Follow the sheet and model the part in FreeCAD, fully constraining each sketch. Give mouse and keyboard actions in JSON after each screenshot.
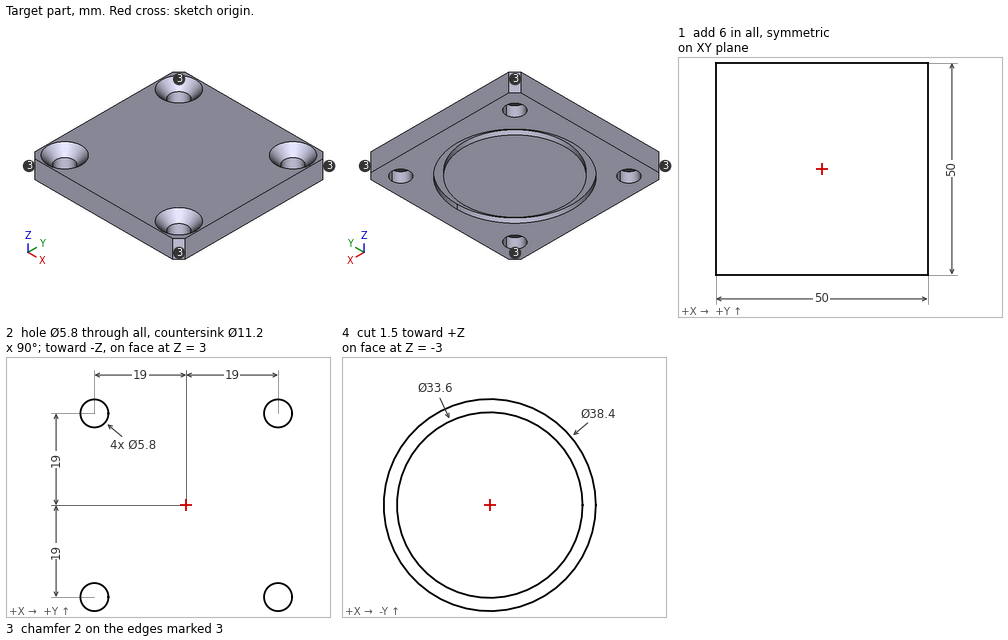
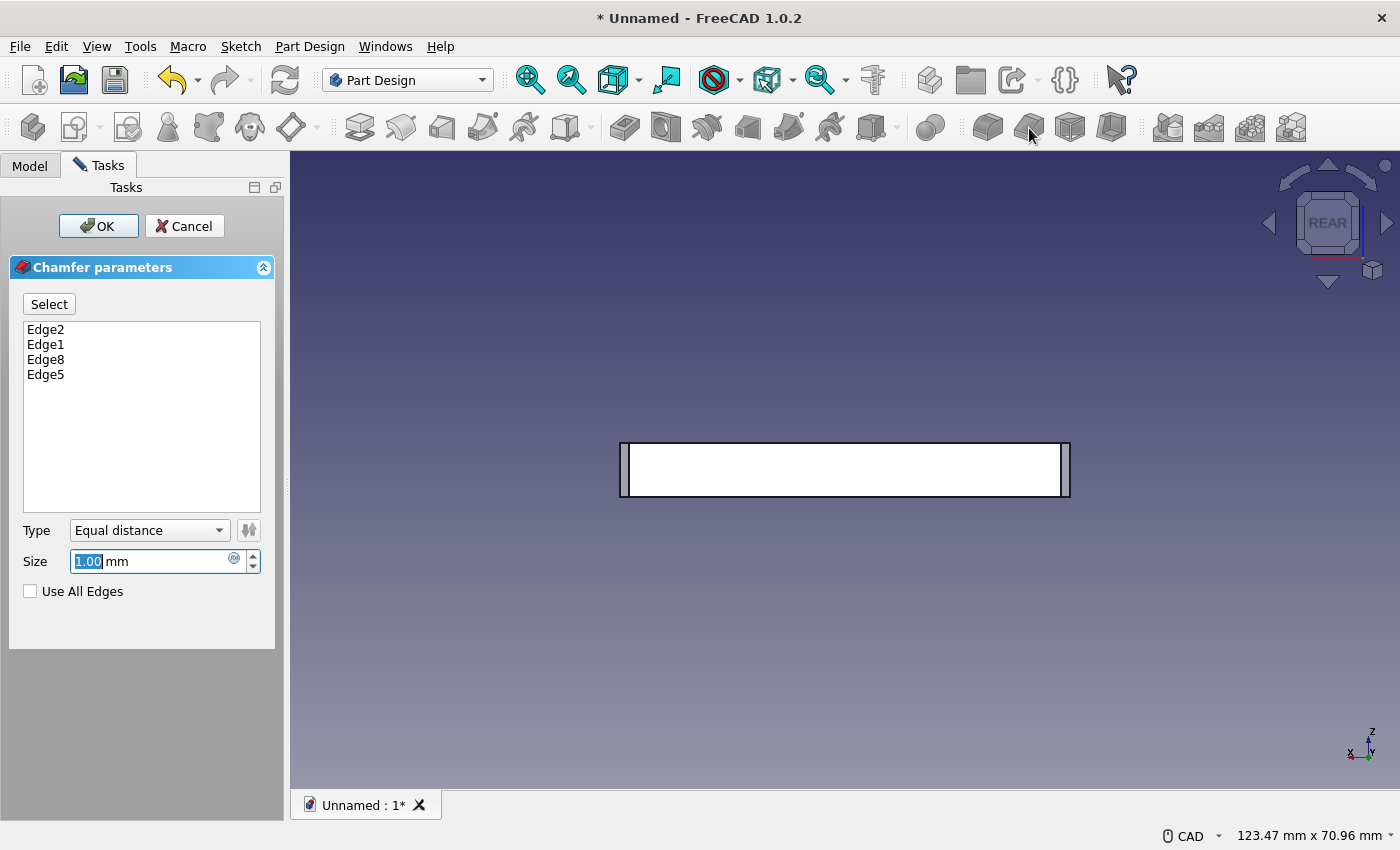
{"action": "type", "text": "2"}
{"action": "key", "text": "Tab"}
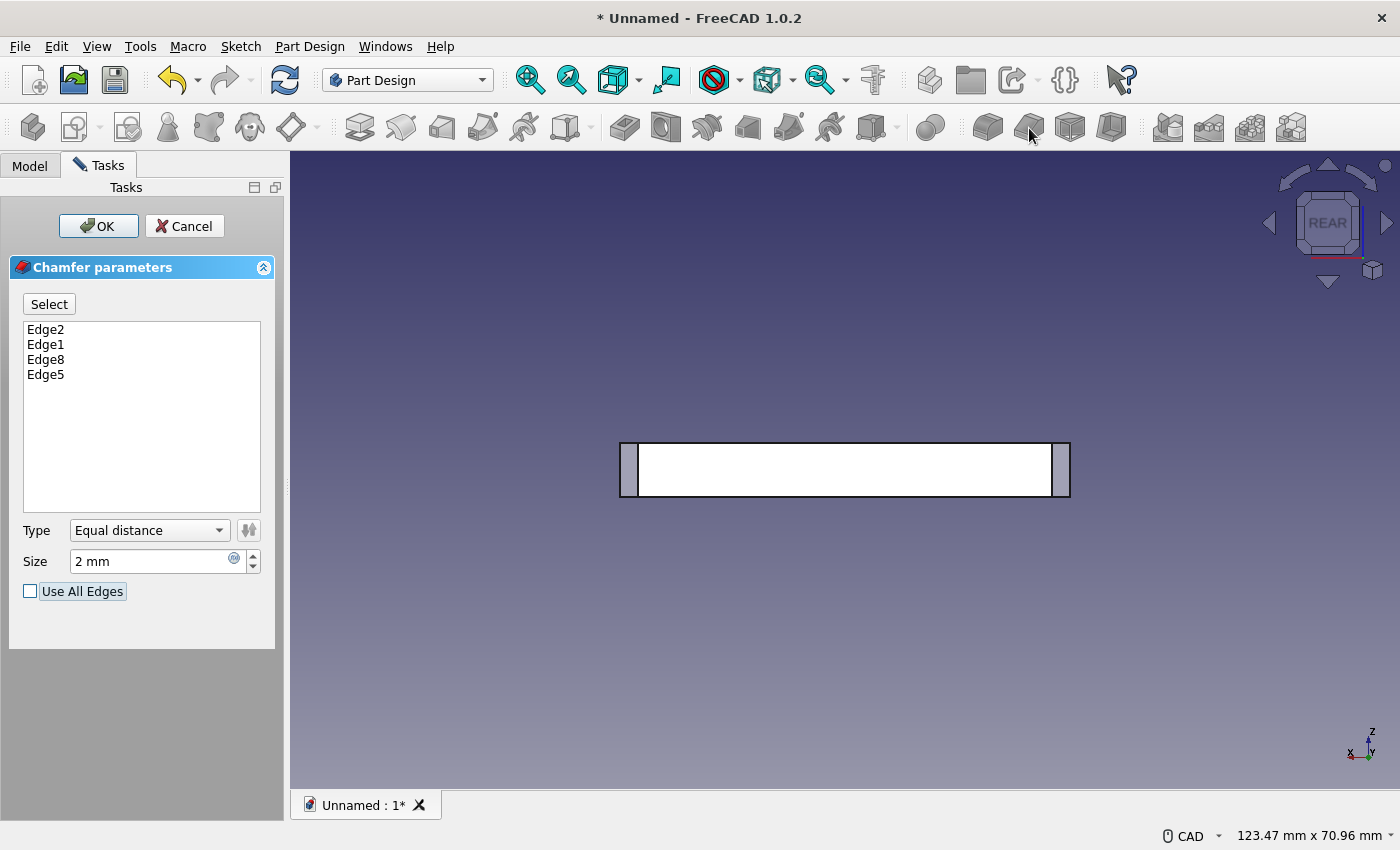
{"action": "left_click", "coordinate": [99, 226]}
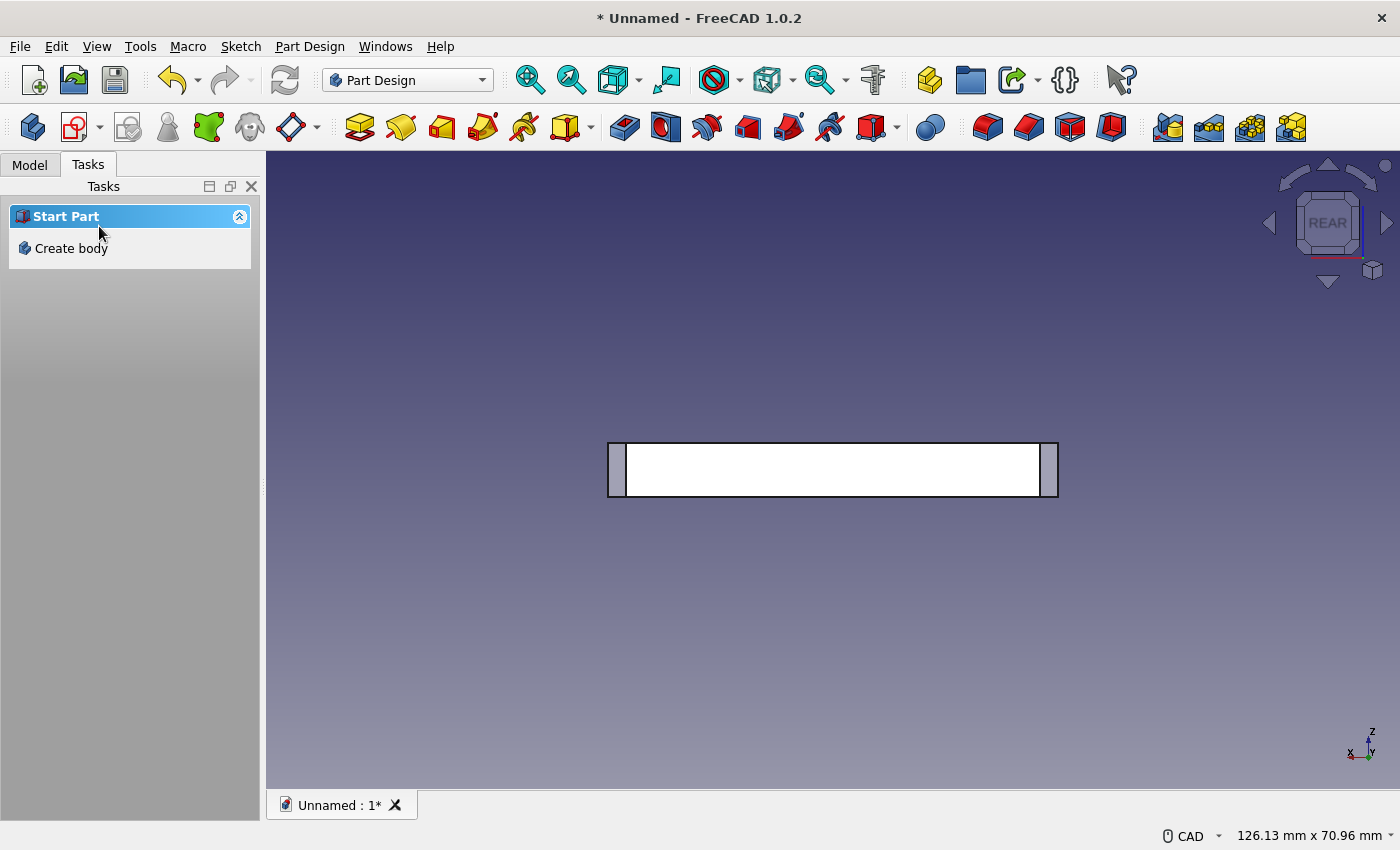
{"action": "left_click", "coordinate": [531, 80]}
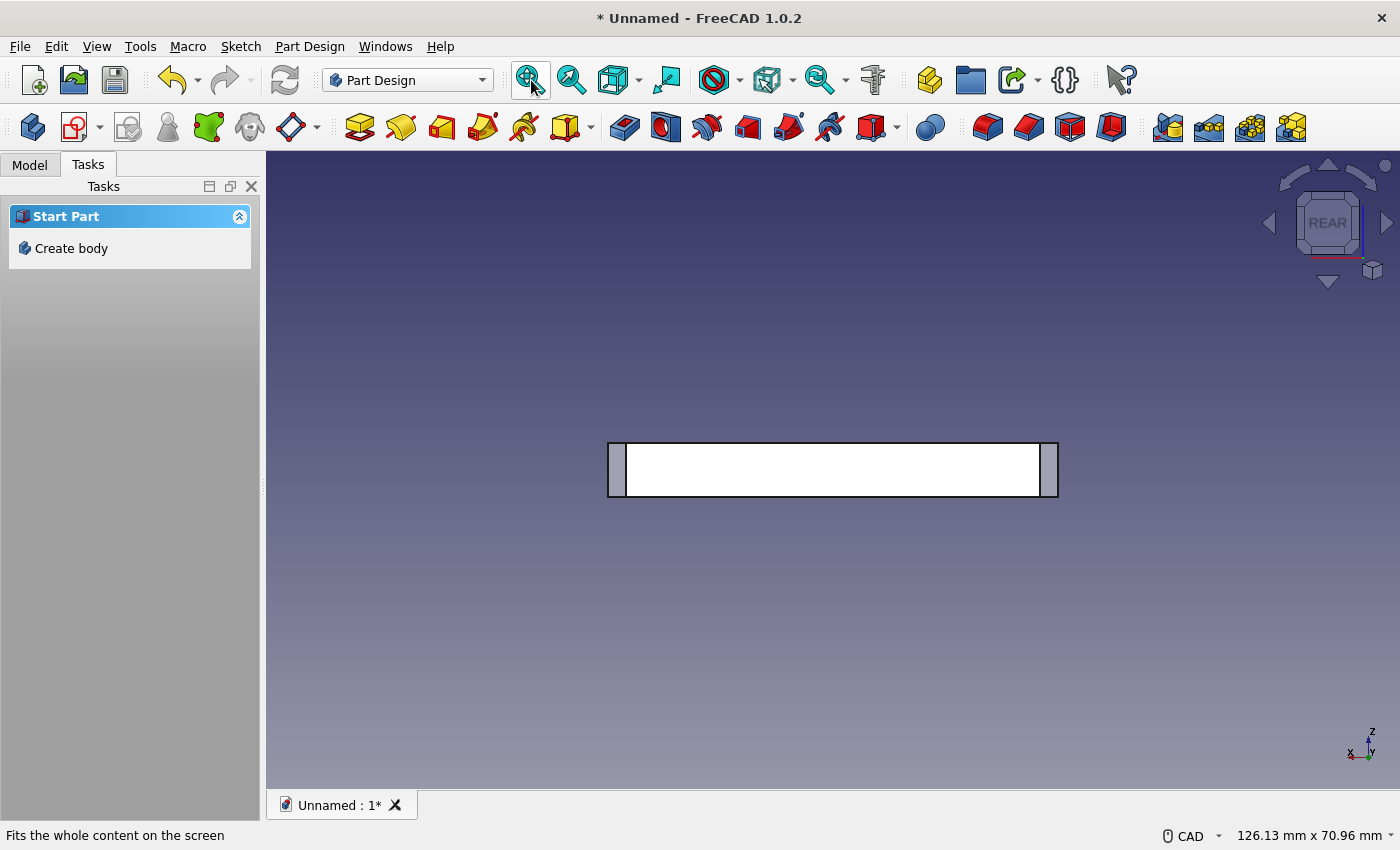
{"action": "key", "text": "5"}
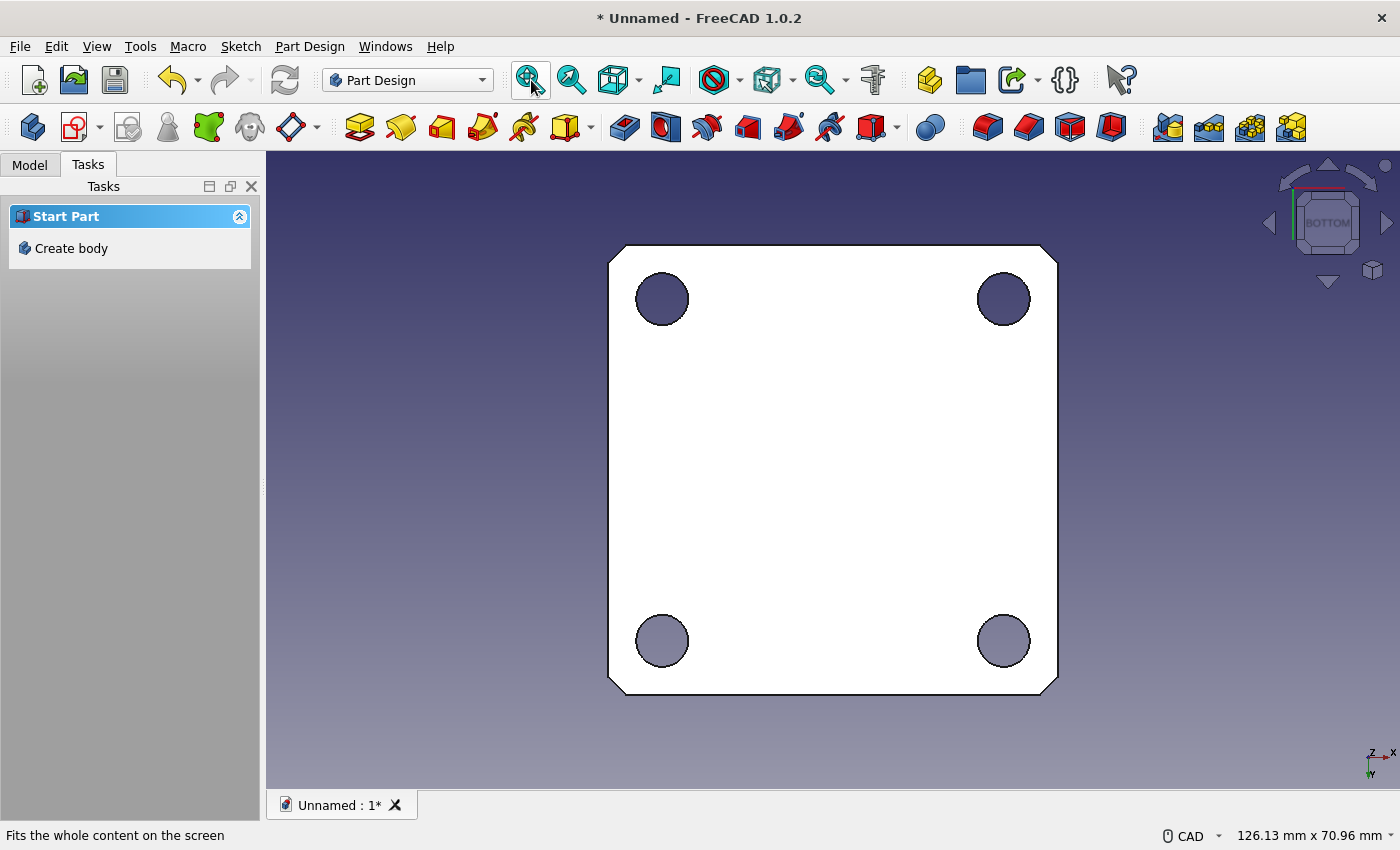
{"action": "left_click", "coordinate": [833, 469]}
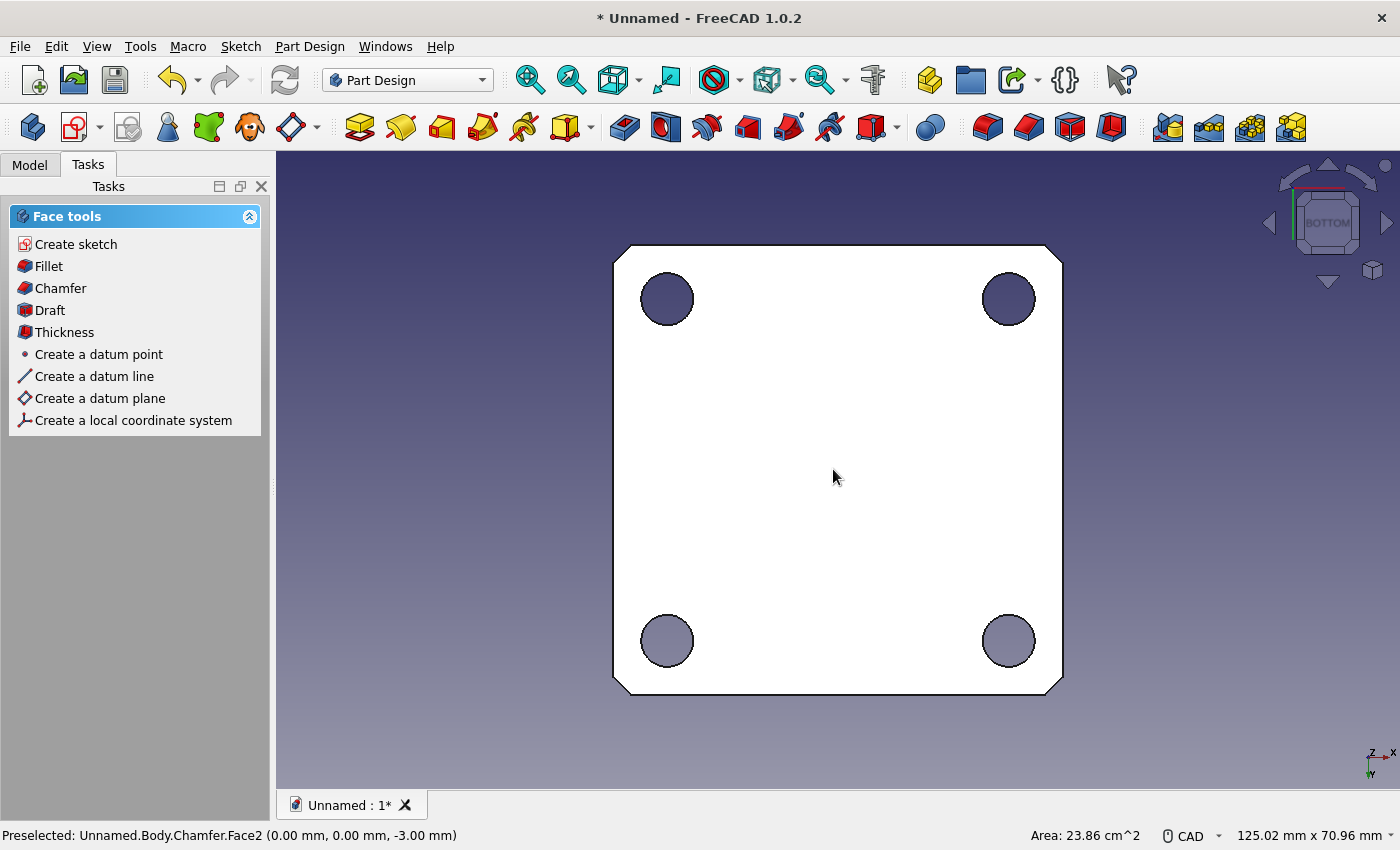
{"action": "left_click", "coordinate": [74, 128]}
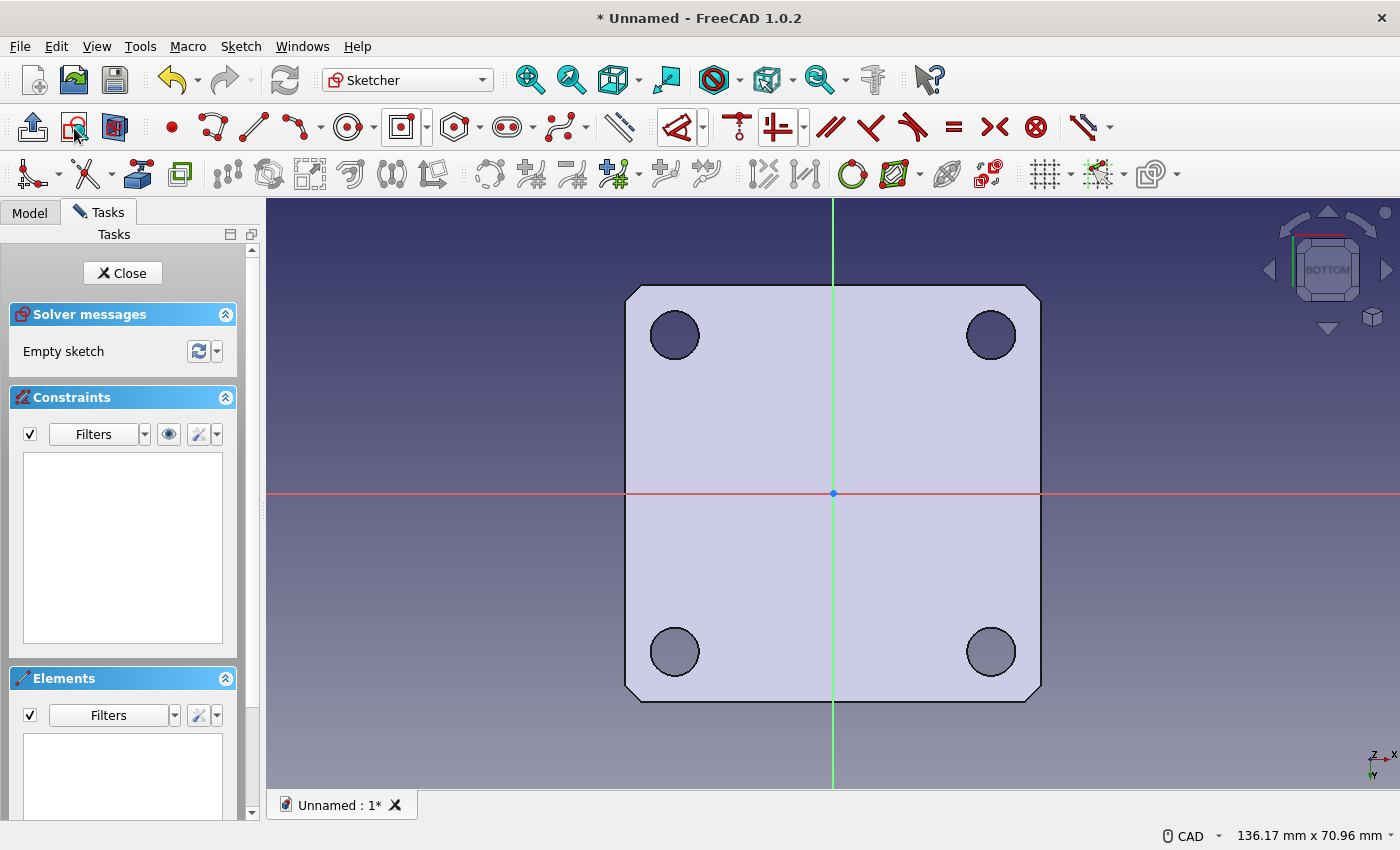
{"action": "left_click", "coordinate": [348, 128]}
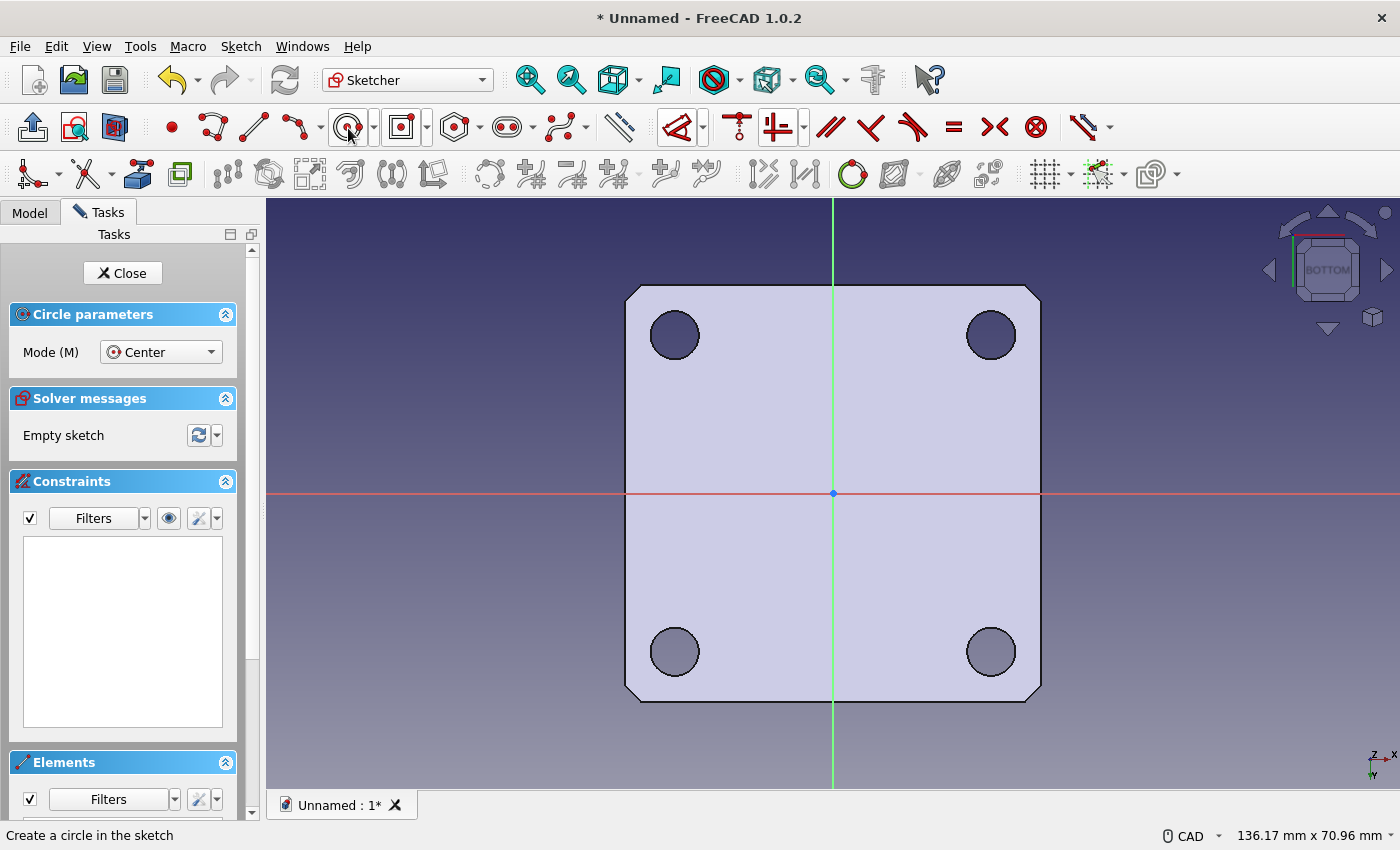
{"action": "left_click", "coordinate": [833, 494]}
{"action": "left_click", "coordinate": [946, 380]}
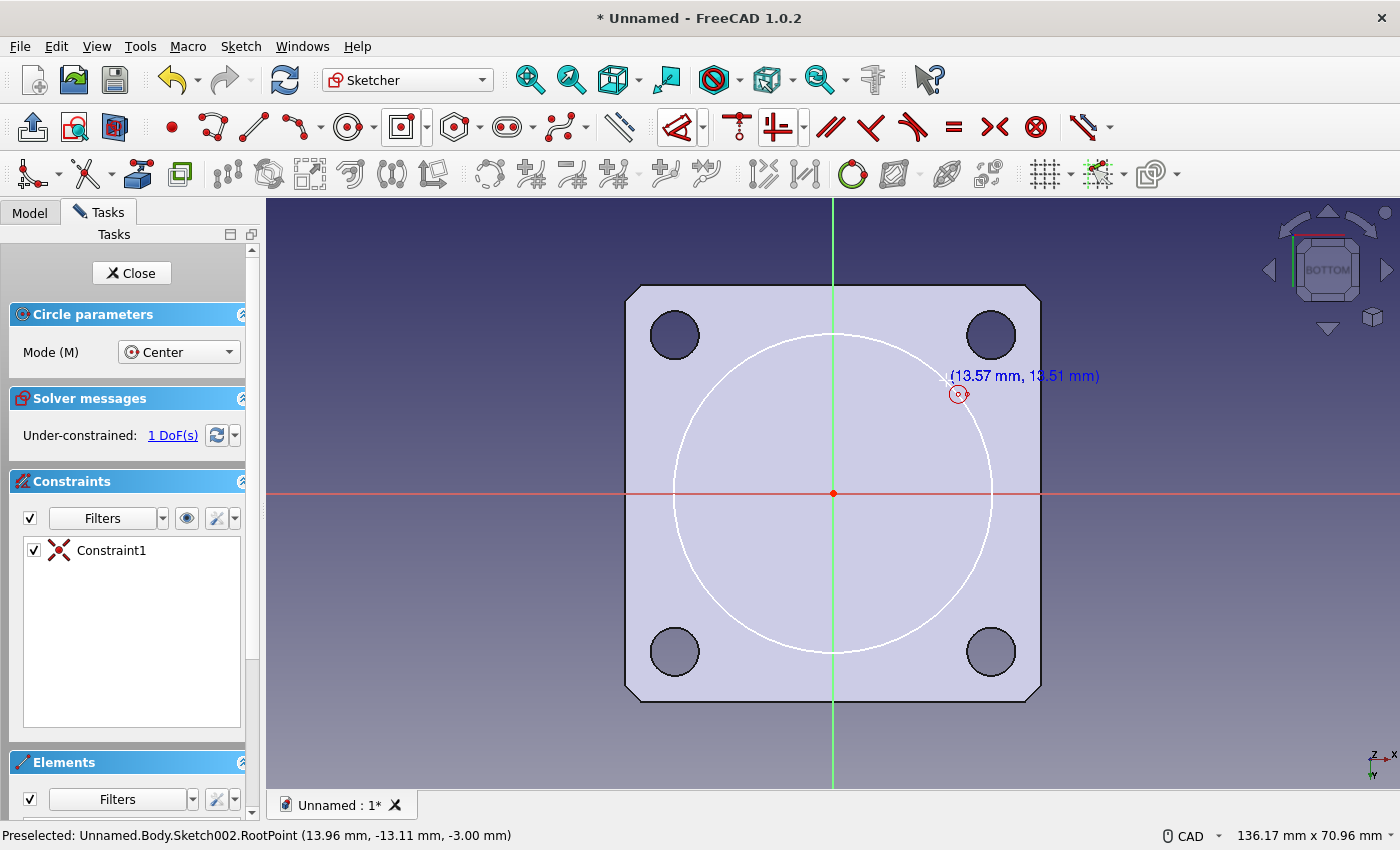
{"action": "left_click", "coordinate": [833, 494]}
{"action": "left_click", "coordinate": [932, 395]}
{"action": "key", "text": "Escape"}